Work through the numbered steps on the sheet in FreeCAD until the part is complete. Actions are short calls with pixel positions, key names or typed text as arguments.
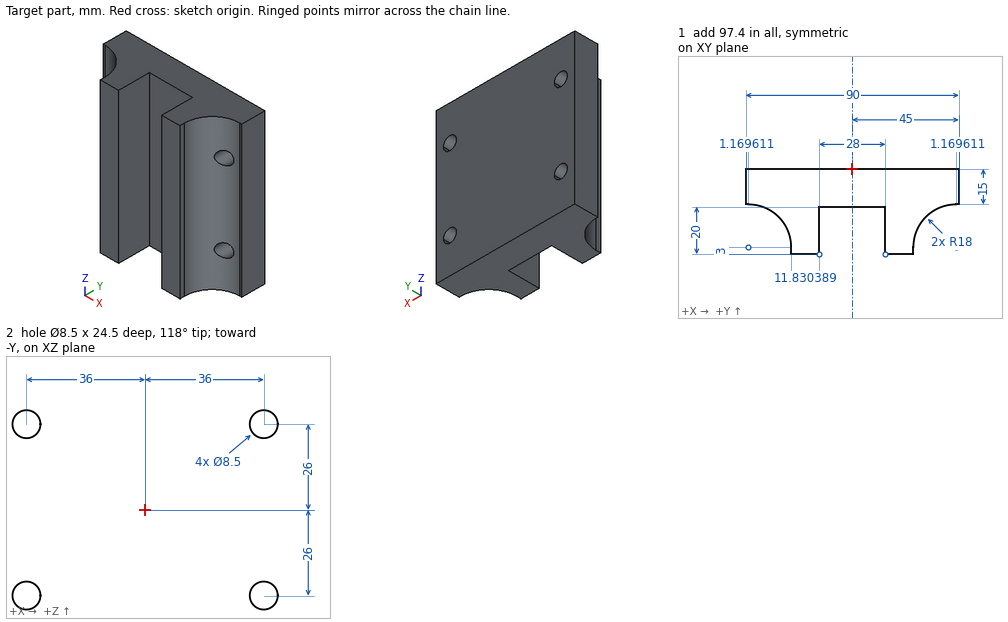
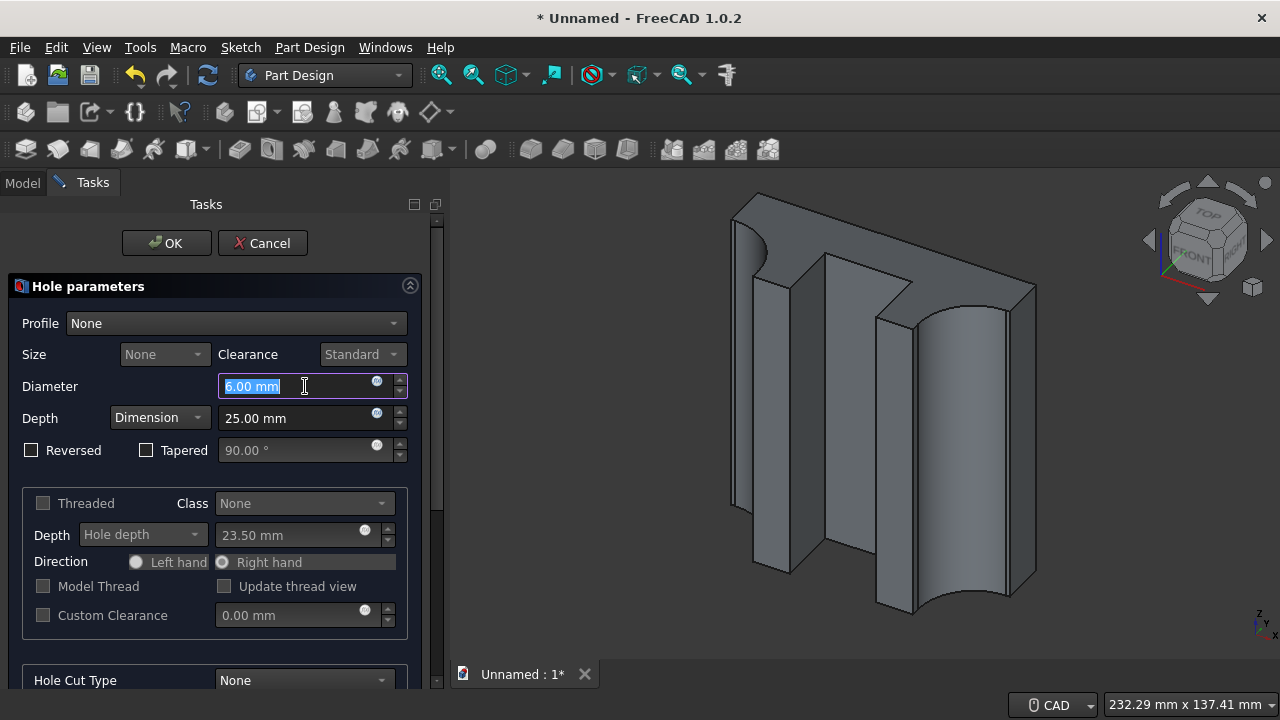
text(8.5)
key(Tab)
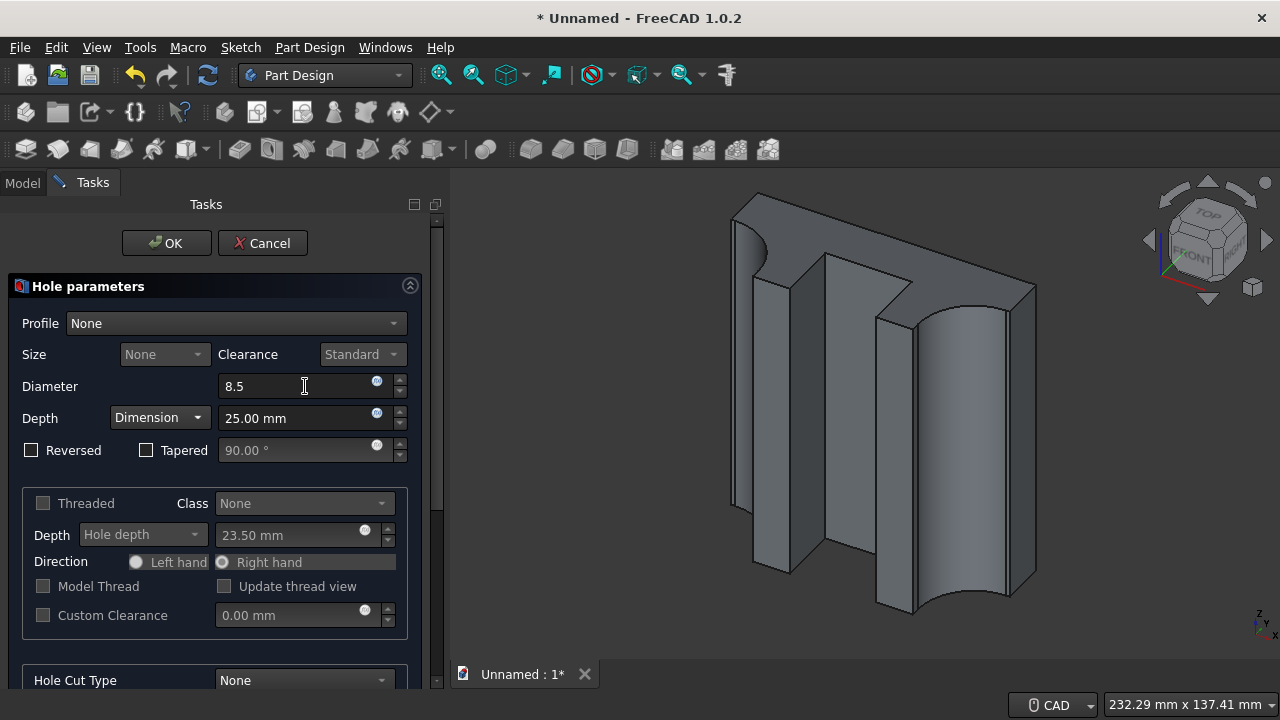
triple_click(305, 418)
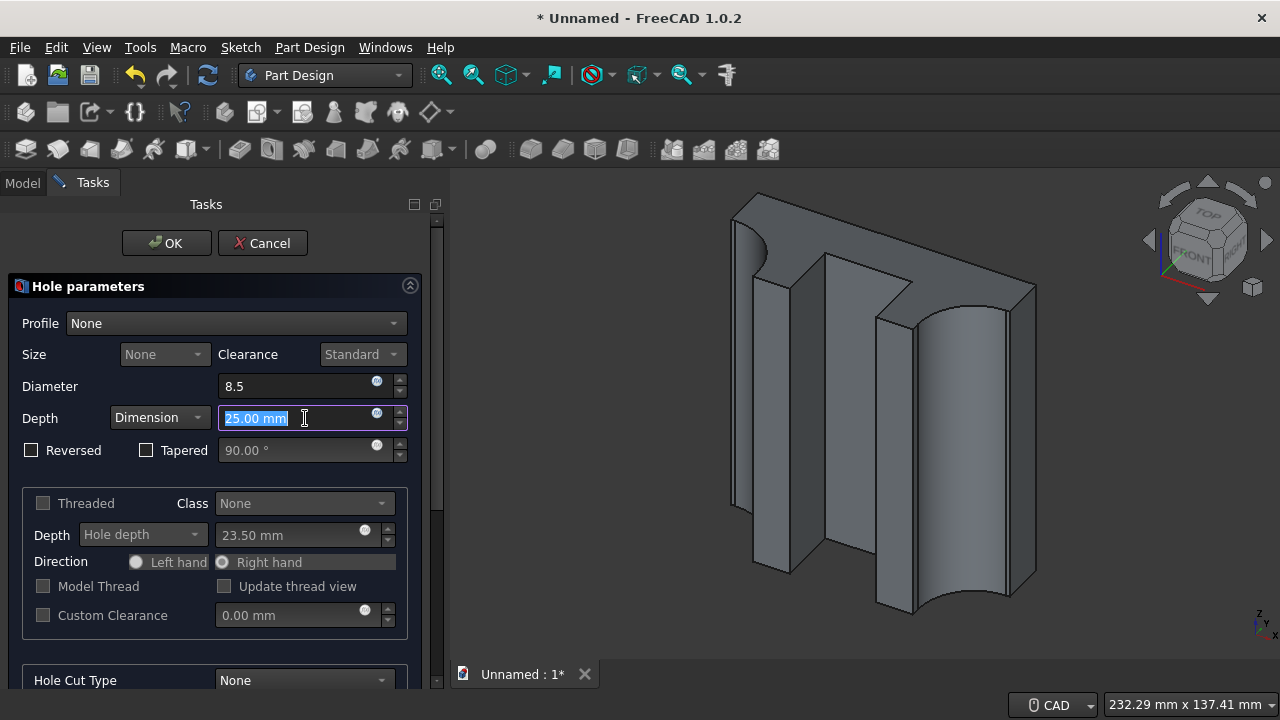
text(24.5)
key(Tab)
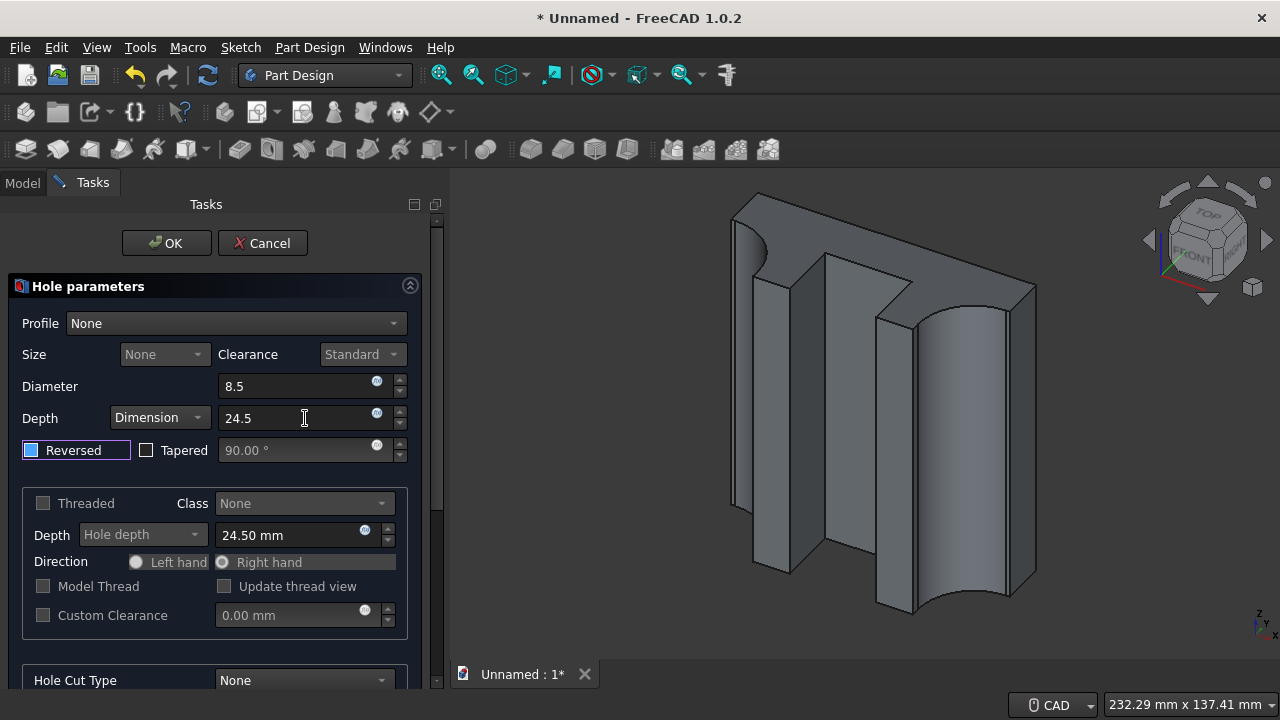
click(30, 450)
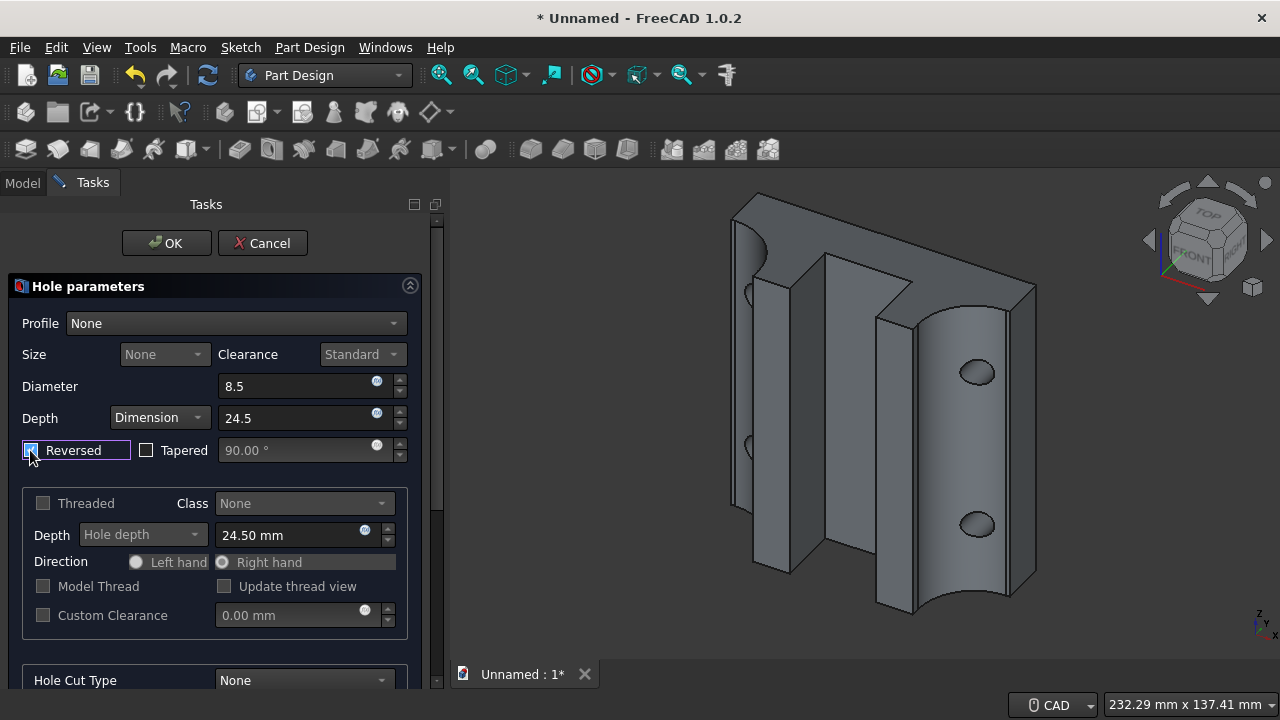
click(167, 243)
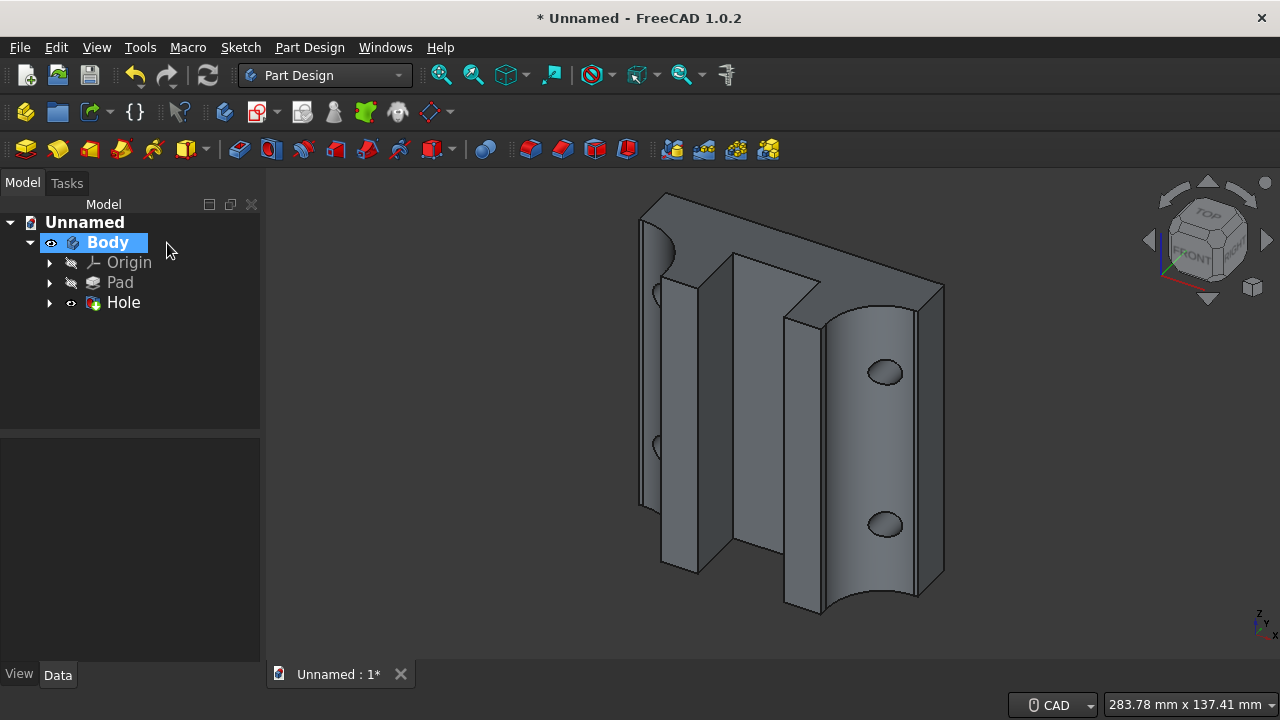
key(0)